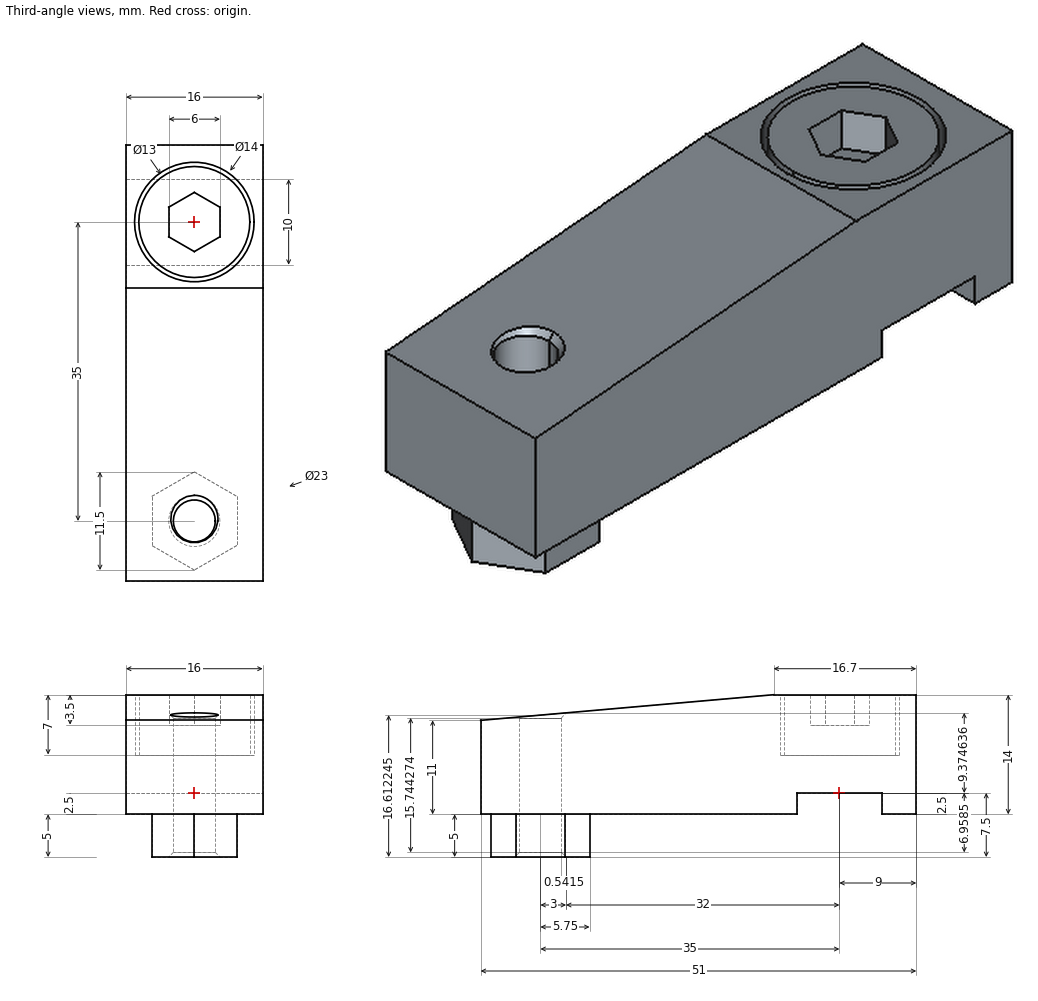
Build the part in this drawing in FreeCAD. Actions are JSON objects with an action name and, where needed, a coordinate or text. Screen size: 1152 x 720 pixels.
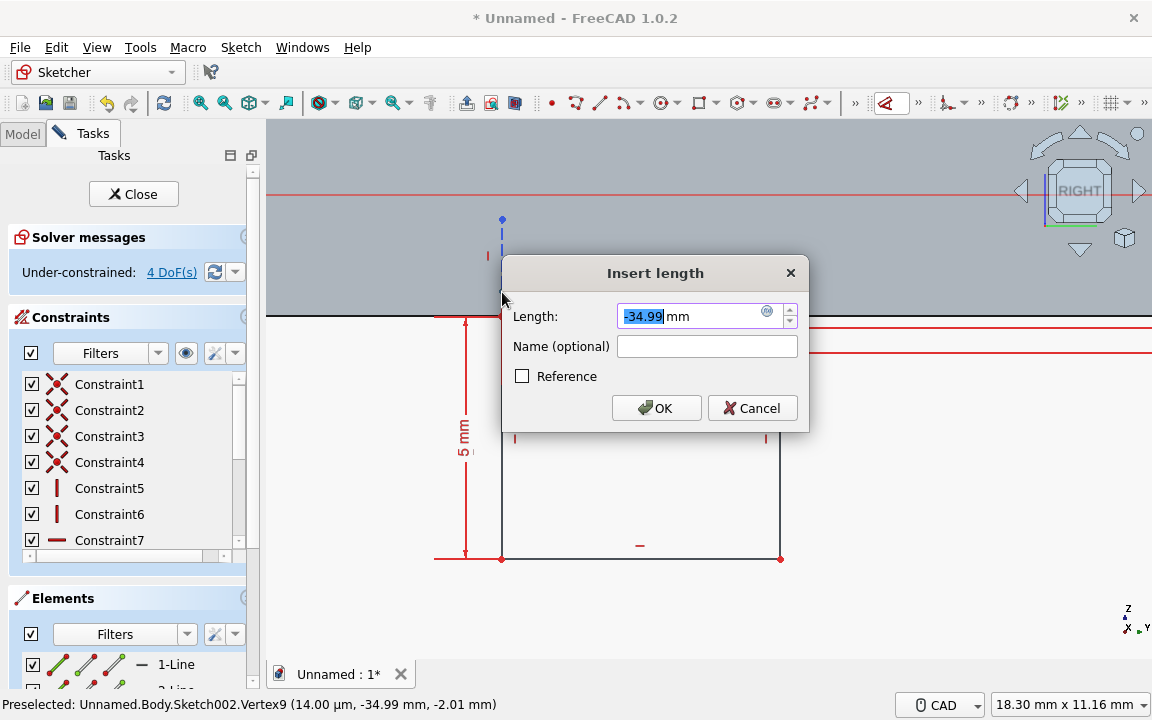
{"action": "type", "text": "-35"}
{"action": "key", "text": "Return"}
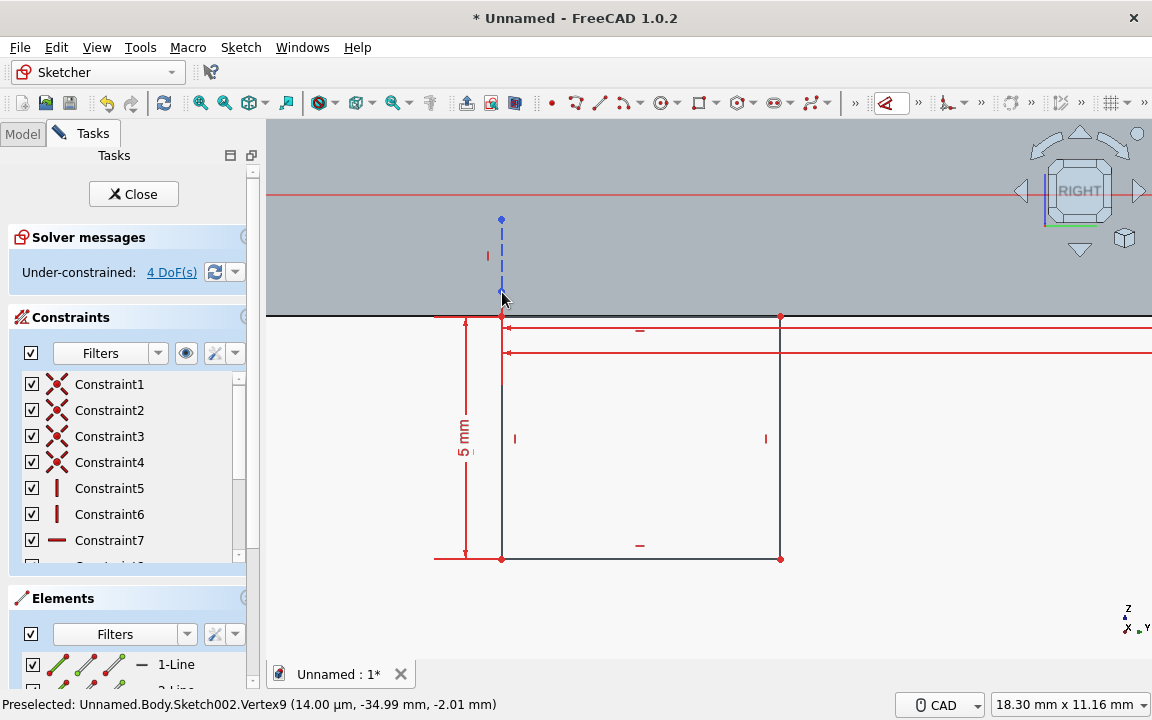
{"action": "left_click", "coordinate": [585, 559]}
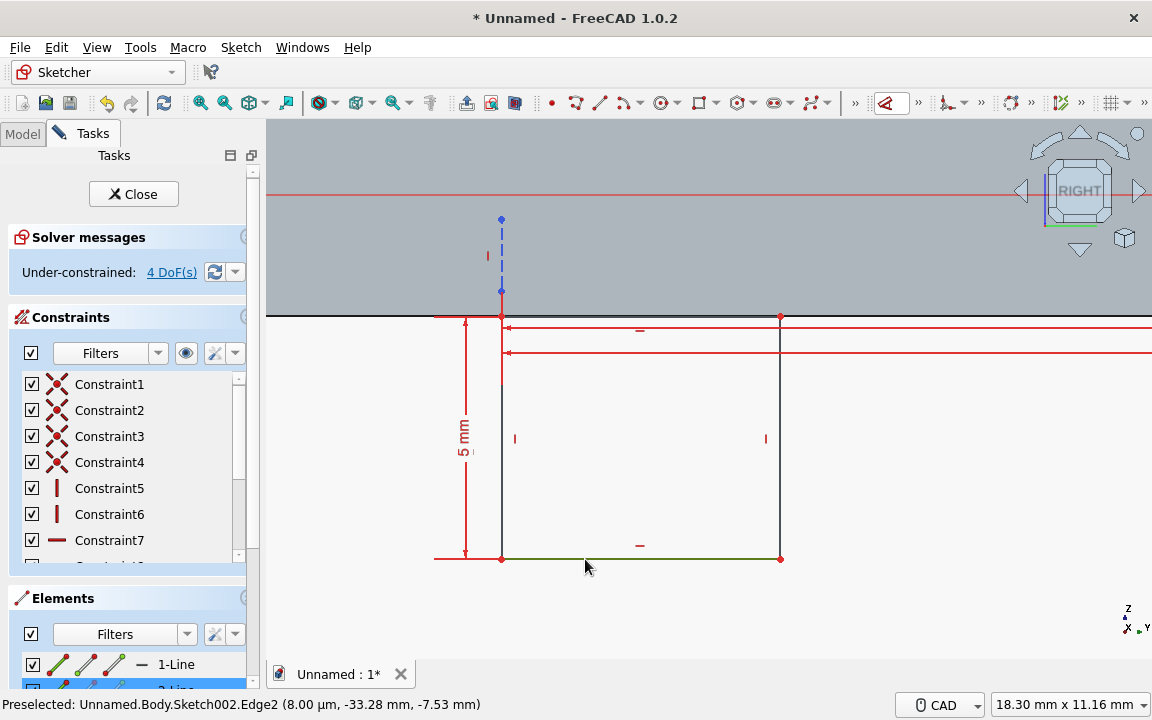
{"action": "key", "text": "l"}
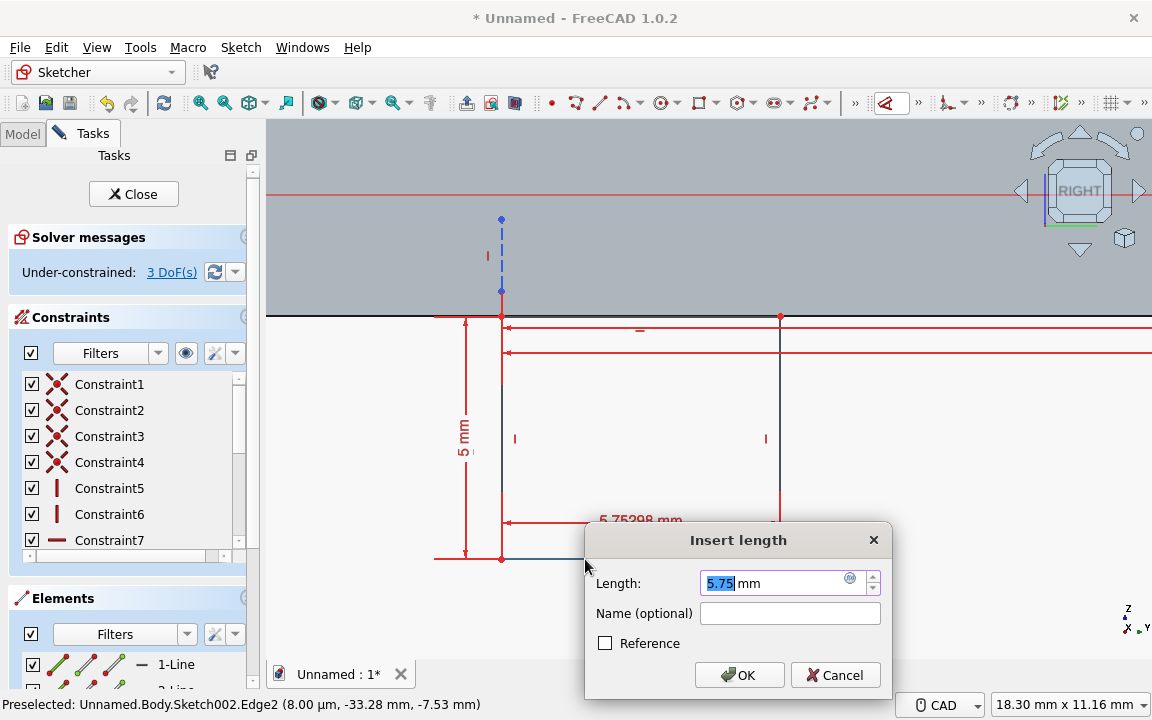
{"action": "type", "text": "5.75"}
{"action": "key", "text": "Return"}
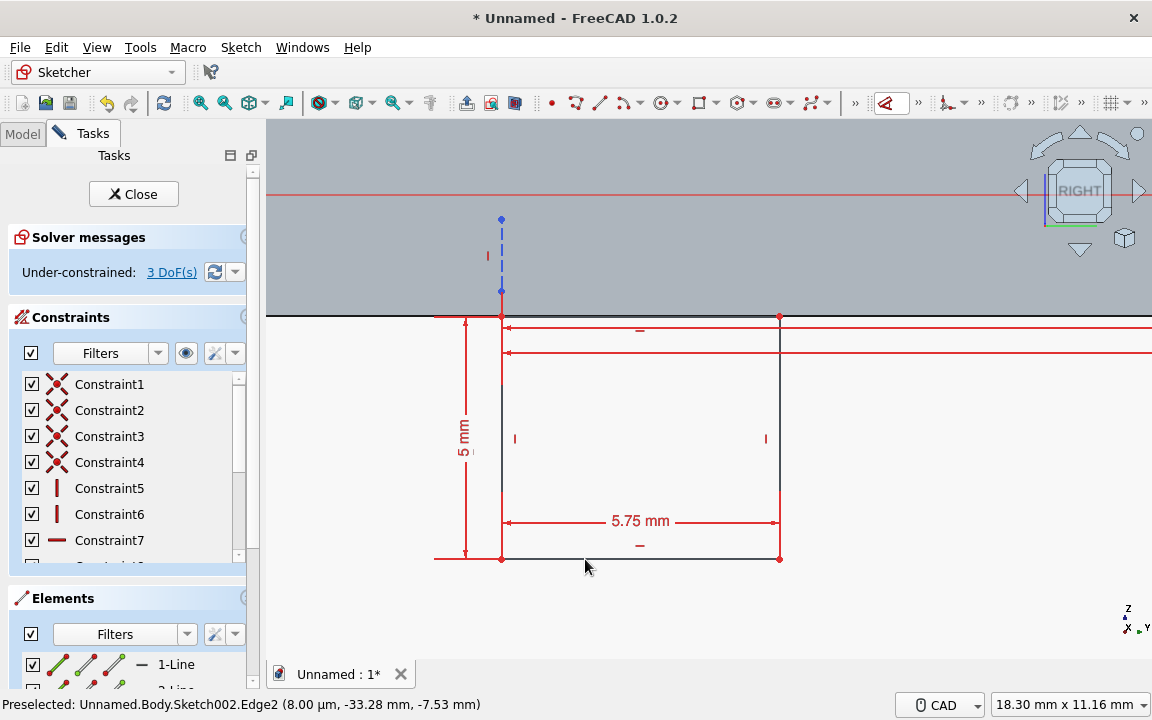
{"action": "left_click", "coordinate": [502, 317]}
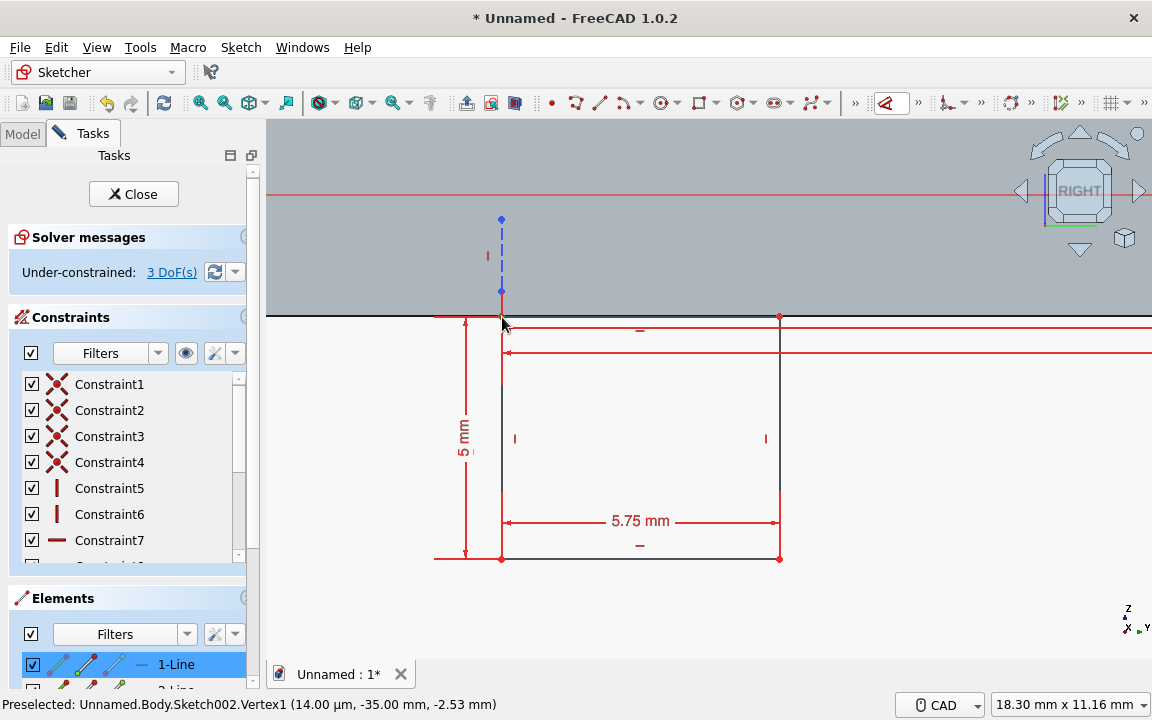
{"action": "key", "text": "i"}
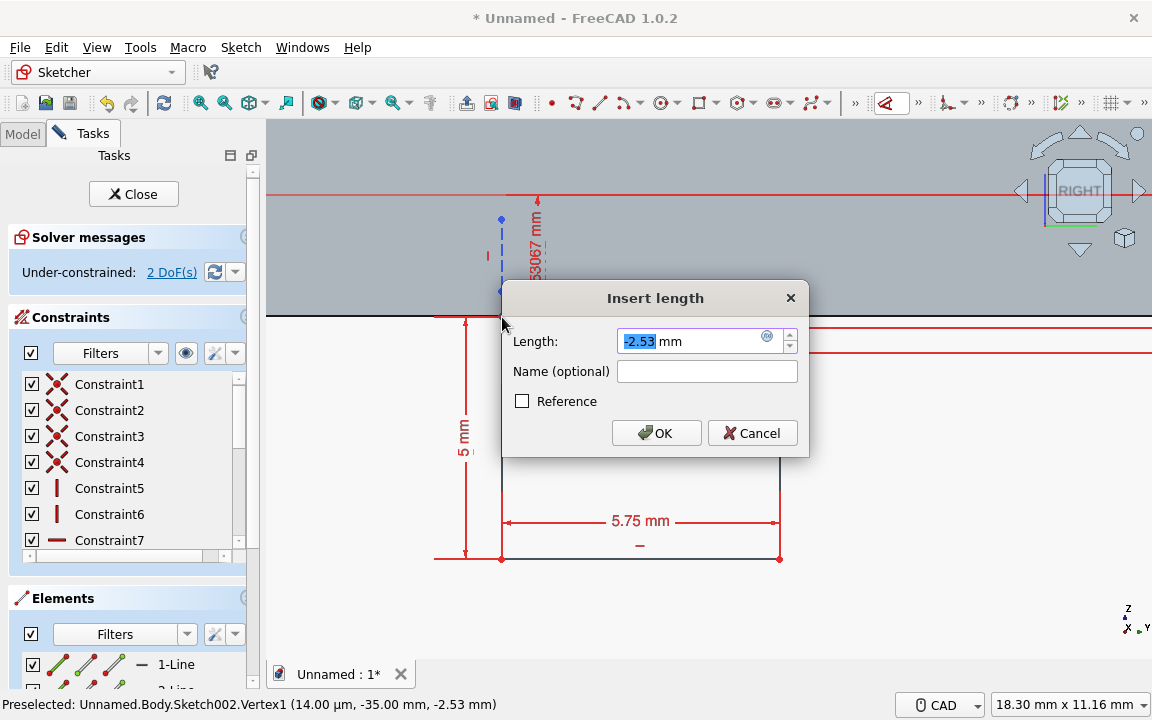
{"action": "type", "text": "-2.5"}
{"action": "key", "text": "Return"}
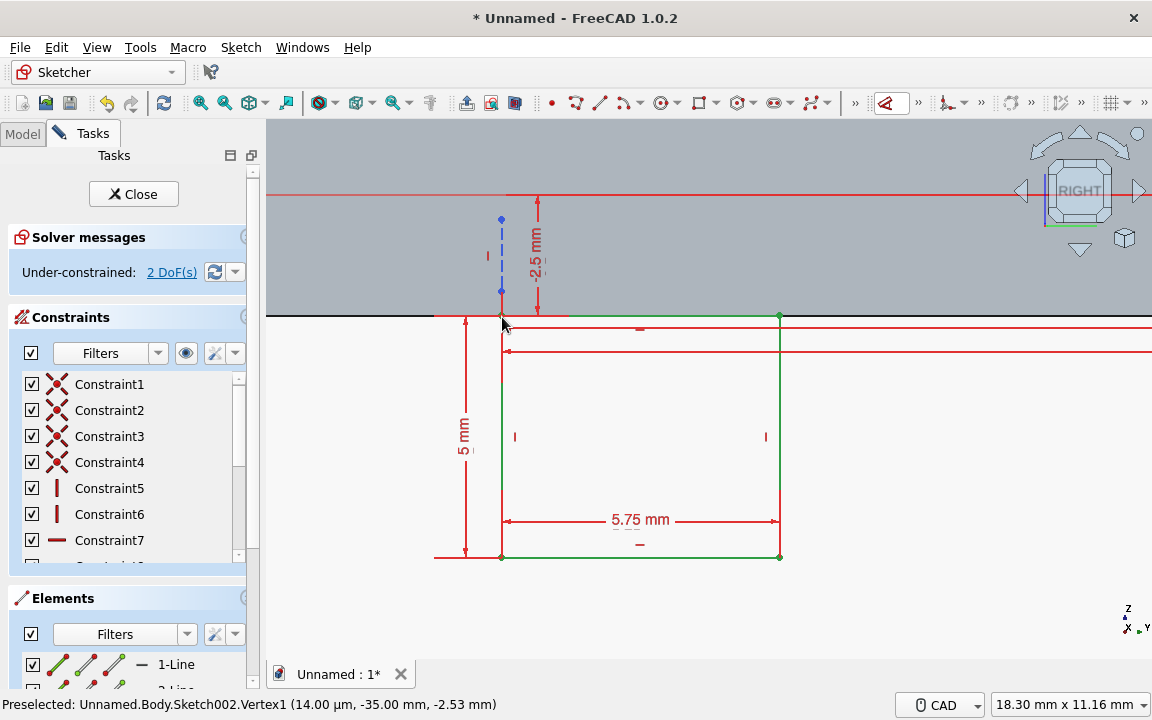
{"action": "left_click", "coordinate": [134, 194]}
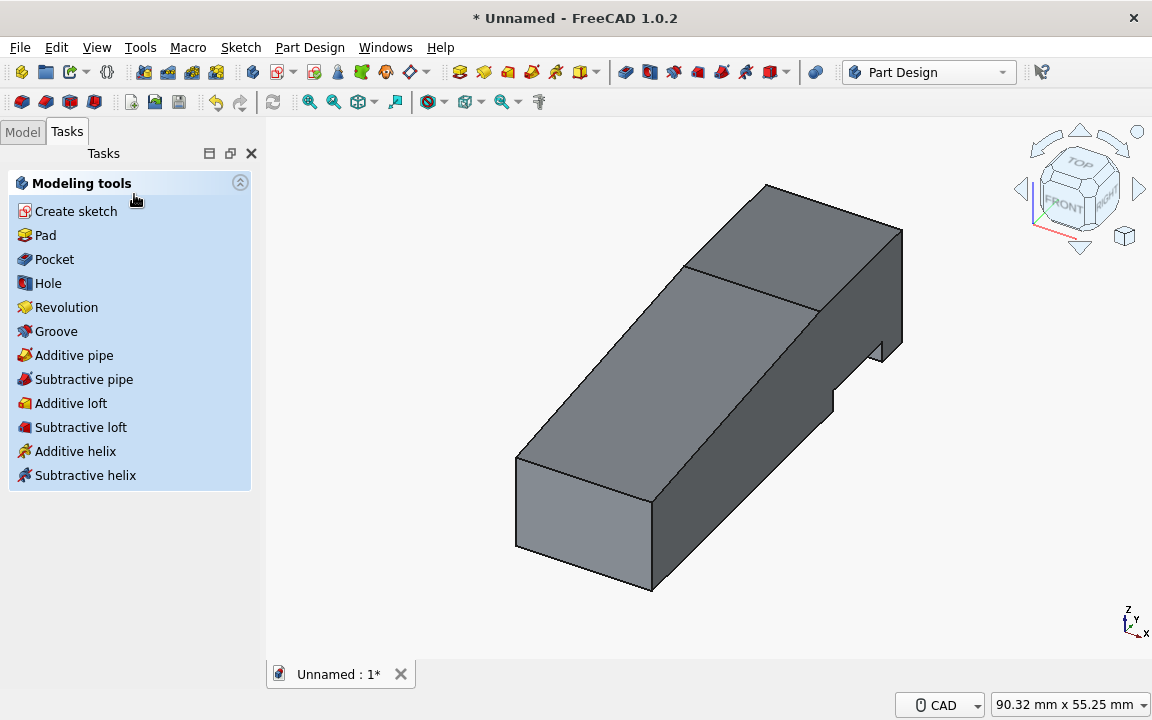
{"action": "left_click", "coordinate": [484, 72]}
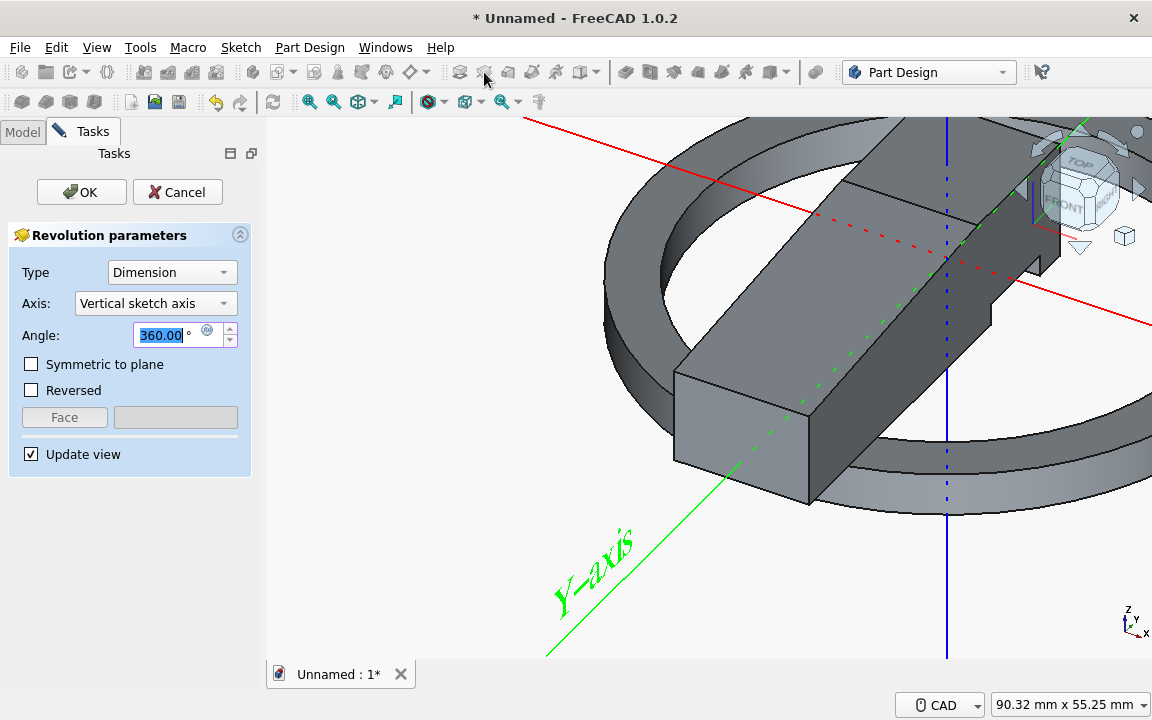
{"action": "left_click", "coordinate": [156, 304]}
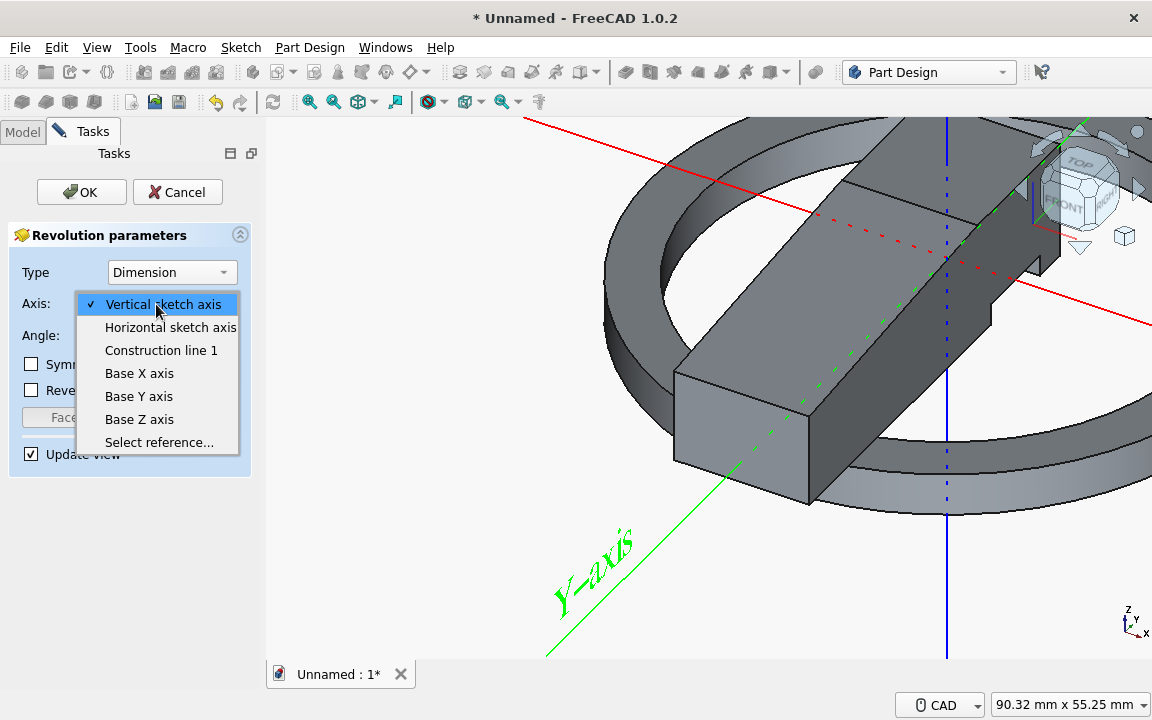
{"action": "left_click", "coordinate": [156, 350]}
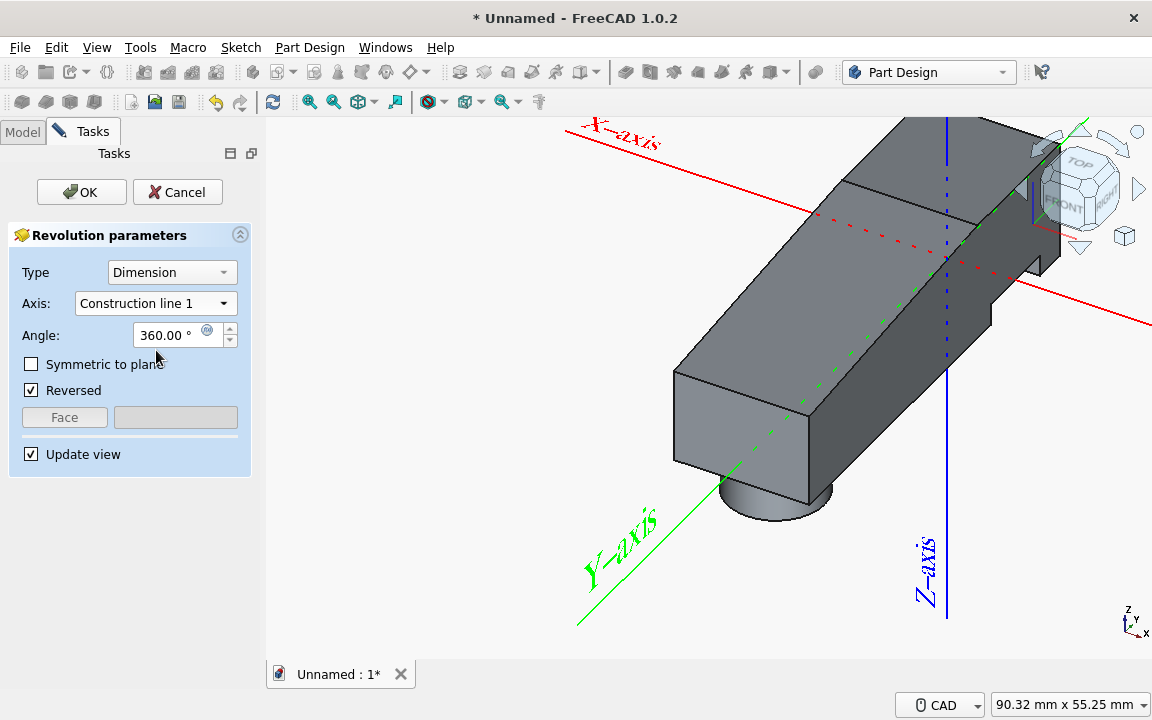
{"action": "left_click", "coordinate": [82, 192]}